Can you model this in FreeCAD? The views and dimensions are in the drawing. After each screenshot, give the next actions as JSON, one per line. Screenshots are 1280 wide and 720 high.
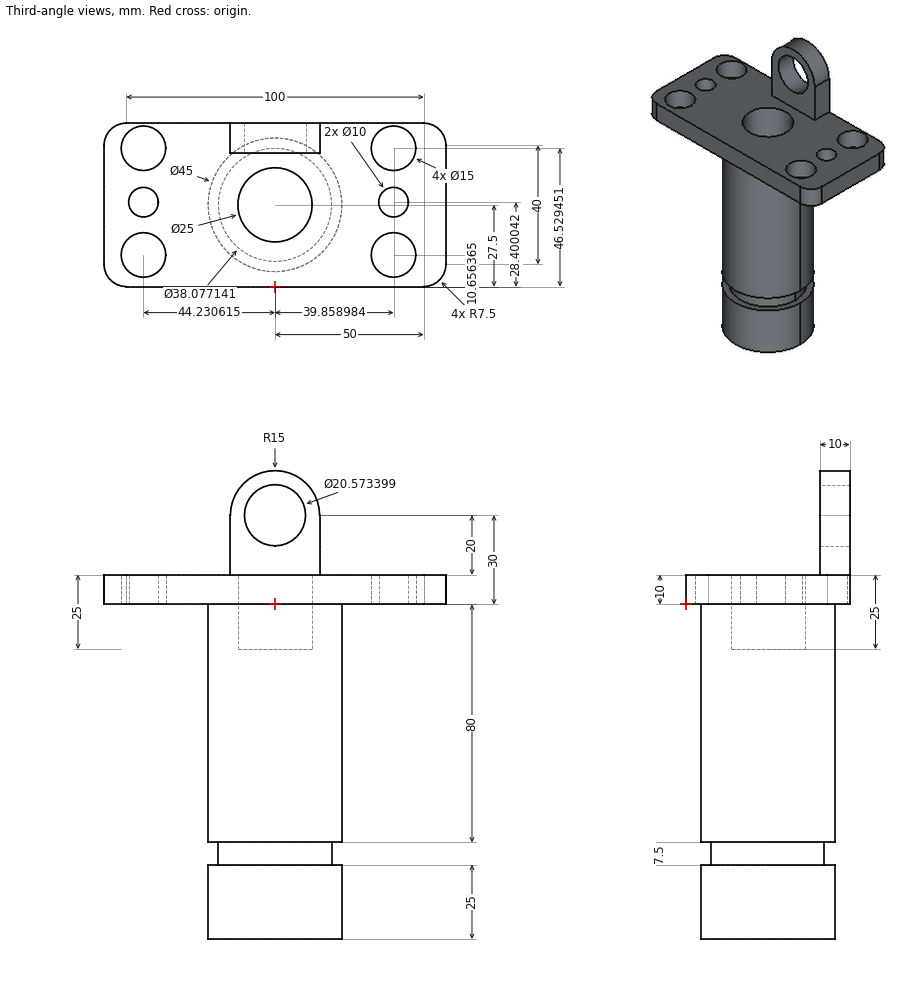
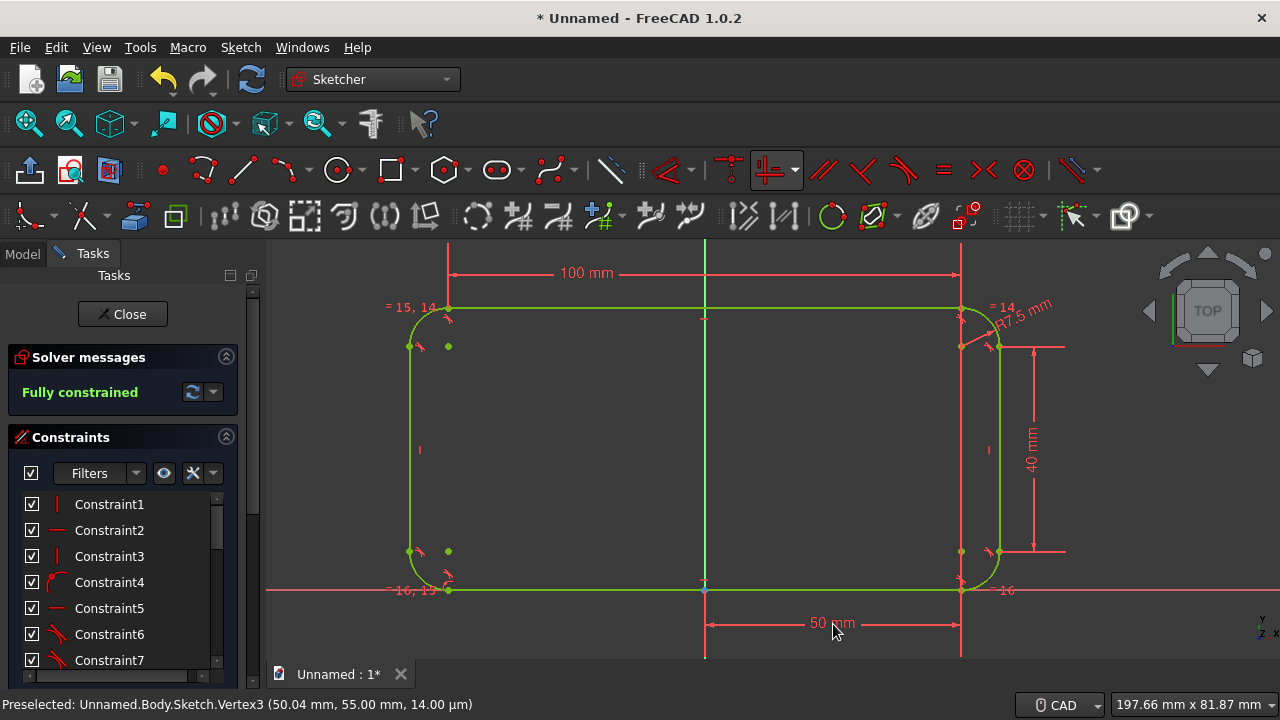
{"action": "left_click", "coordinate": [123, 314]}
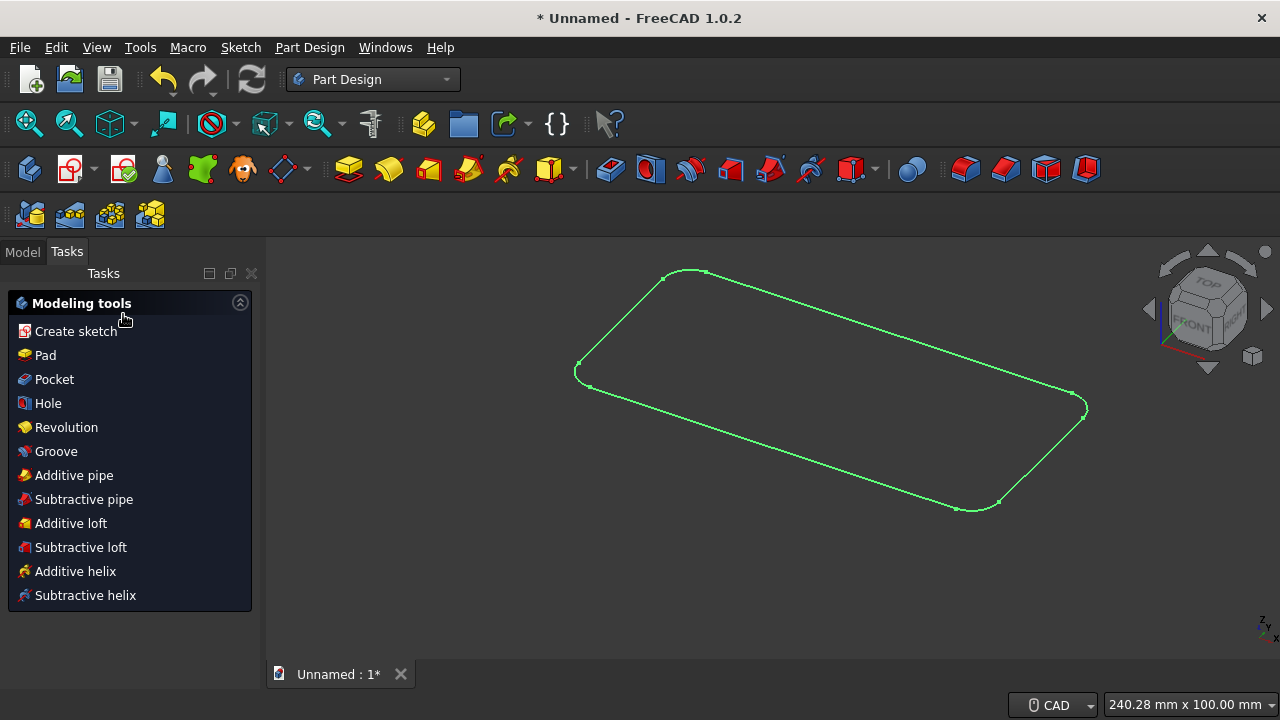
{"action": "left_click", "coordinate": [350, 170]}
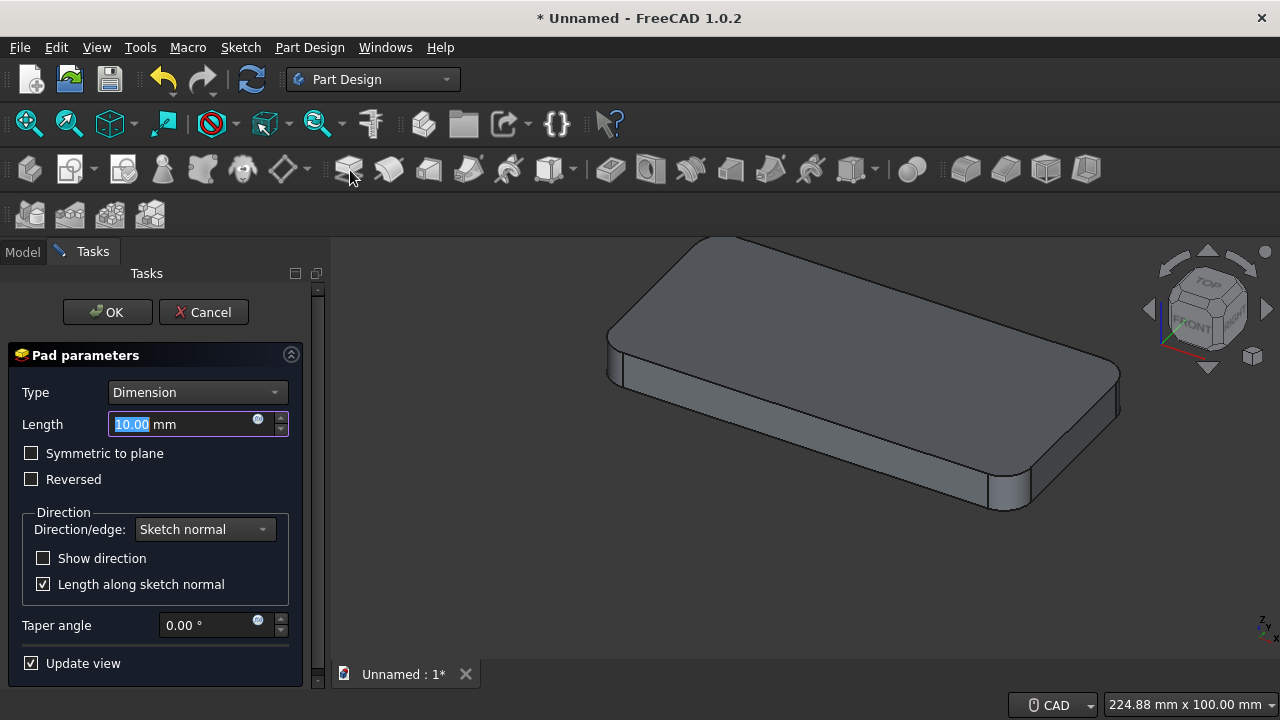
{"action": "type", "text": "10"}
{"action": "key", "text": "Tab"}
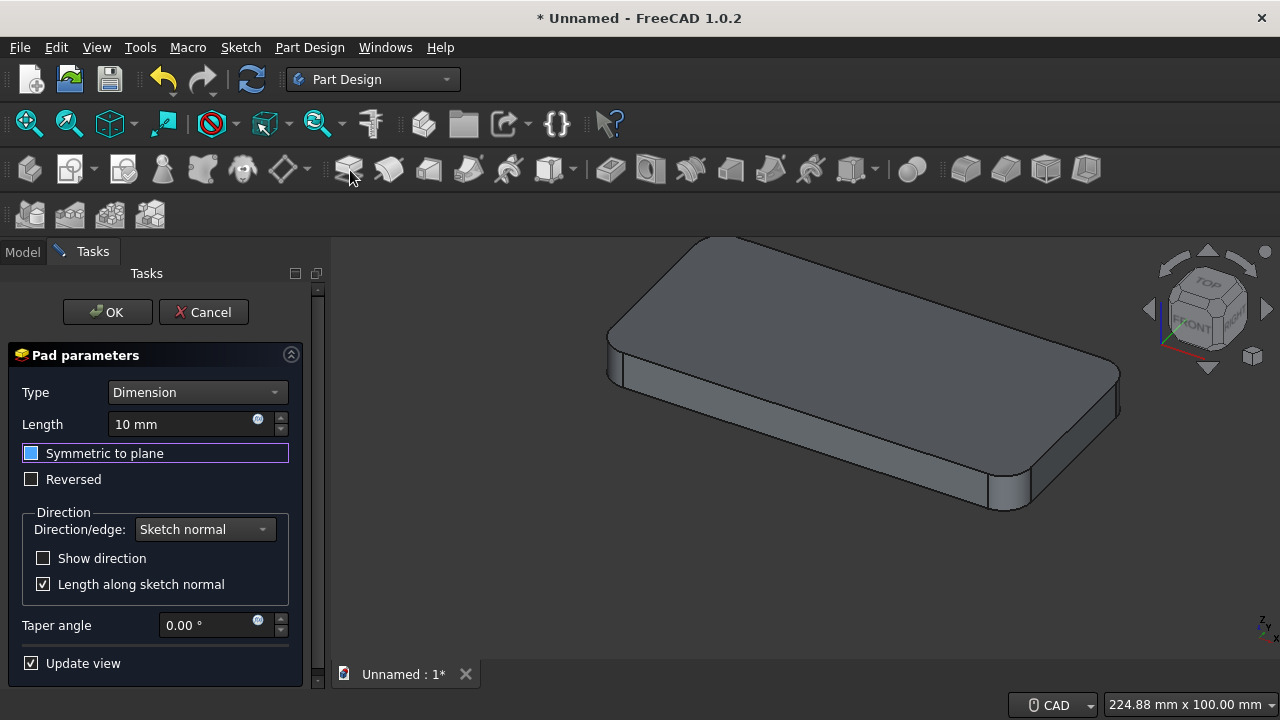
{"action": "left_click", "coordinate": [108, 312]}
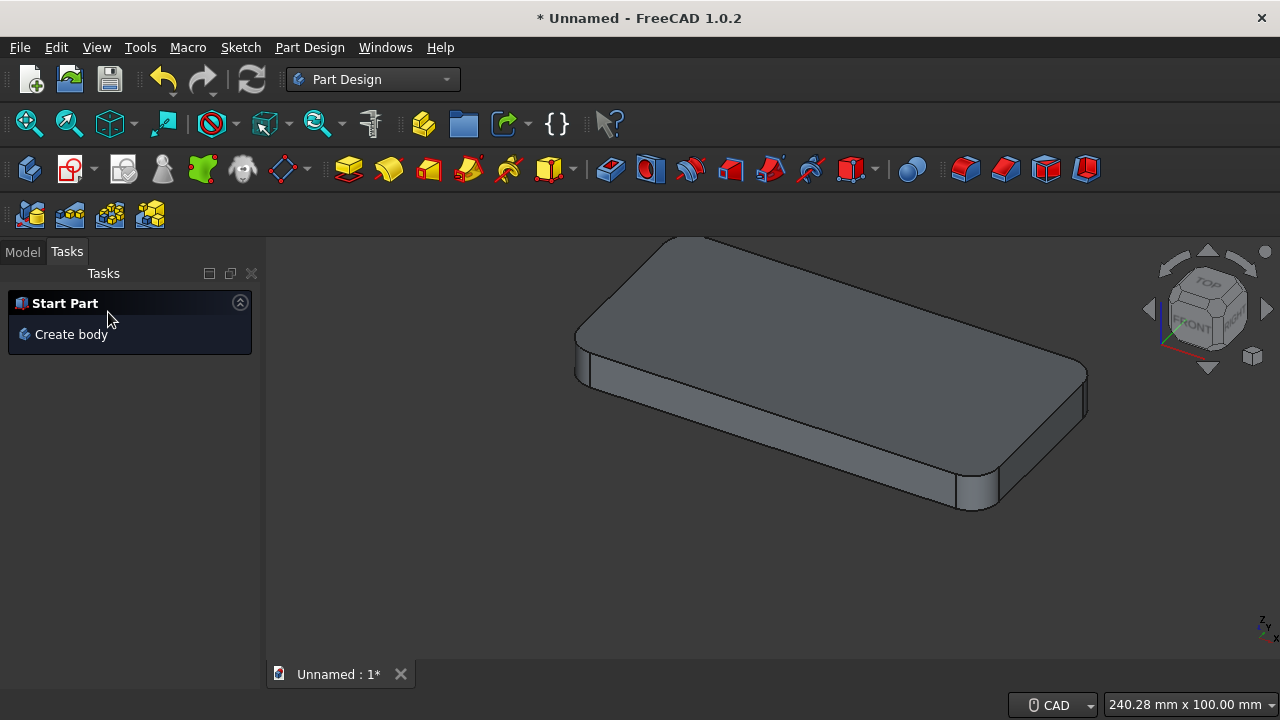
{"action": "left_click", "coordinate": [30, 124]}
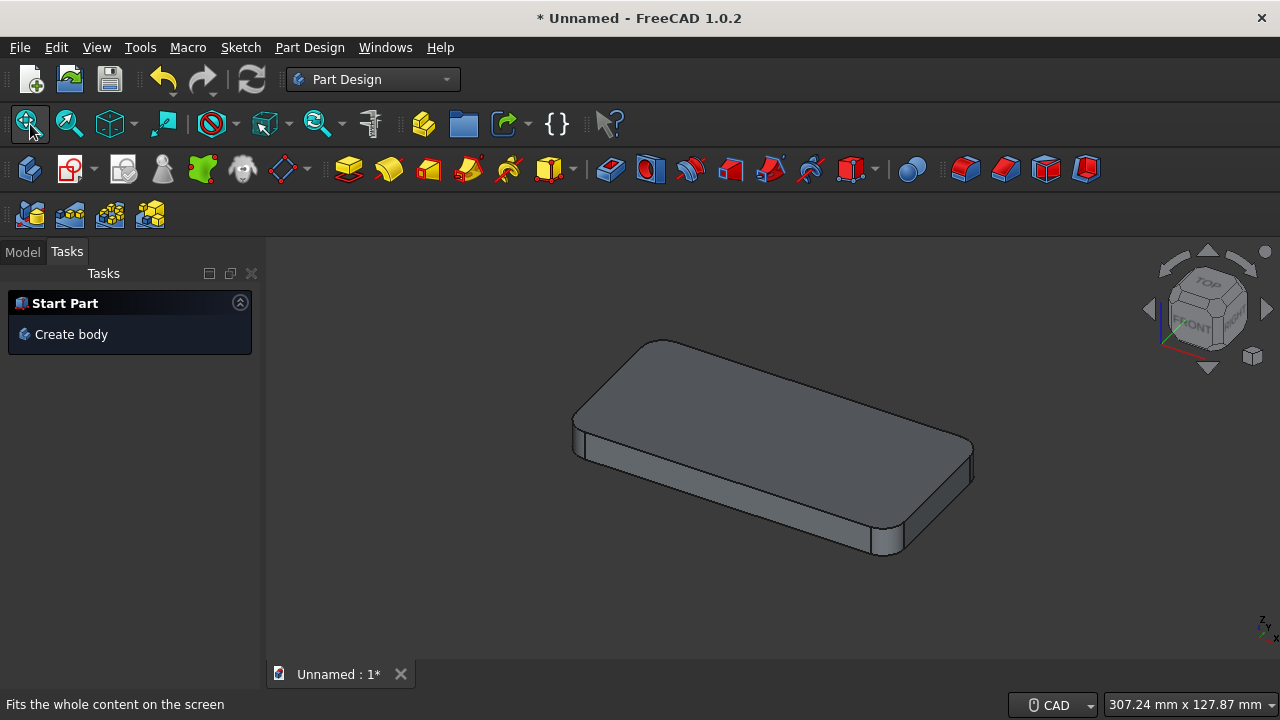
{"action": "key", "text": "5"}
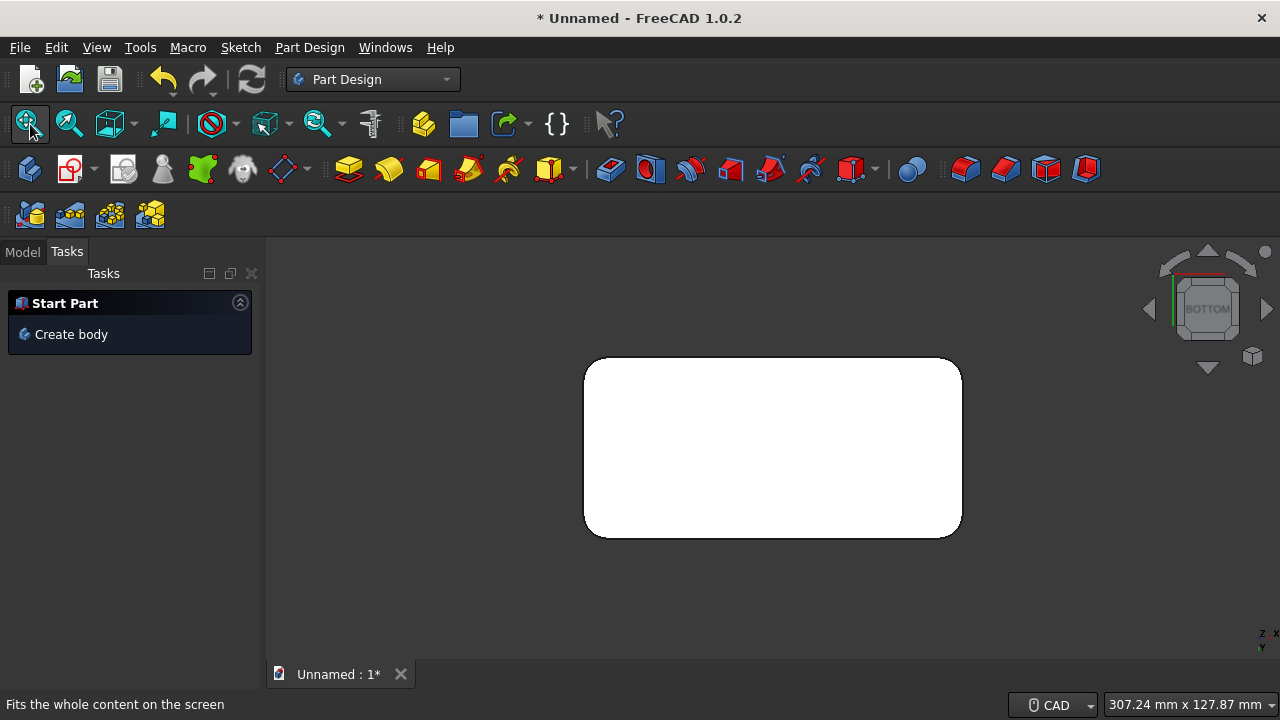
{"action": "left_click", "coordinate": [30, 124]}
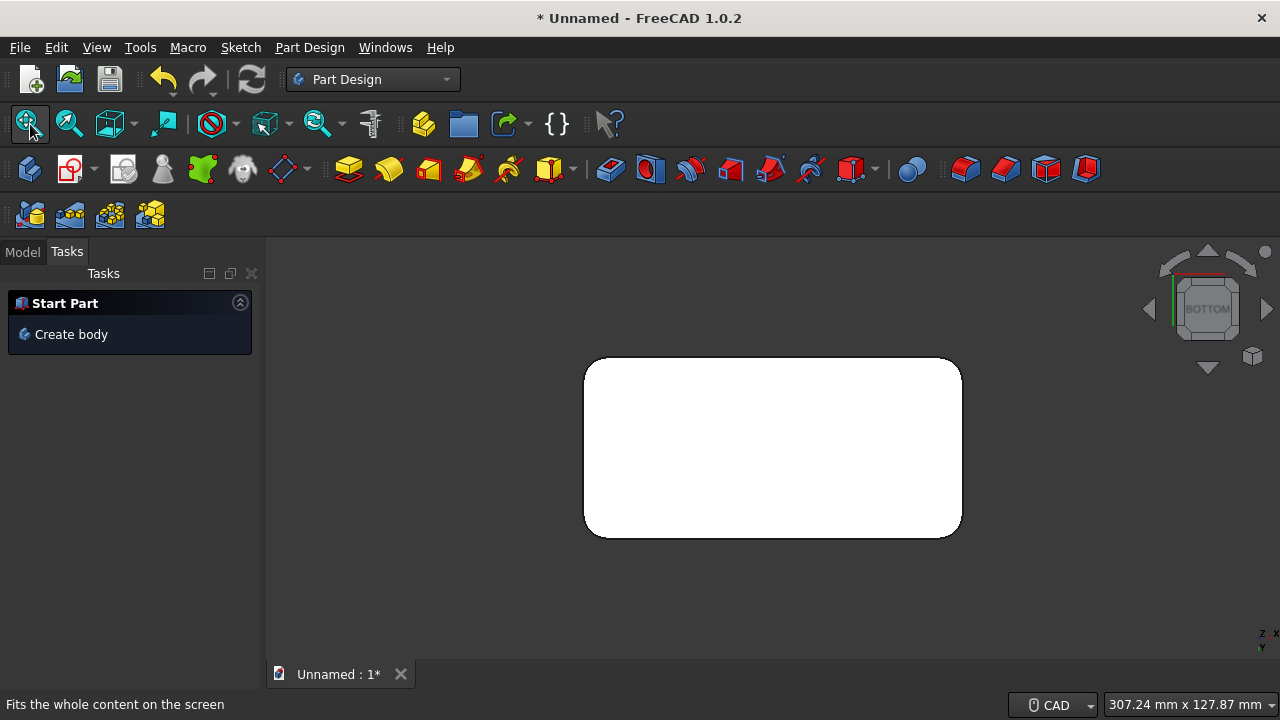
{"action": "left_click", "coordinate": [827, 447]}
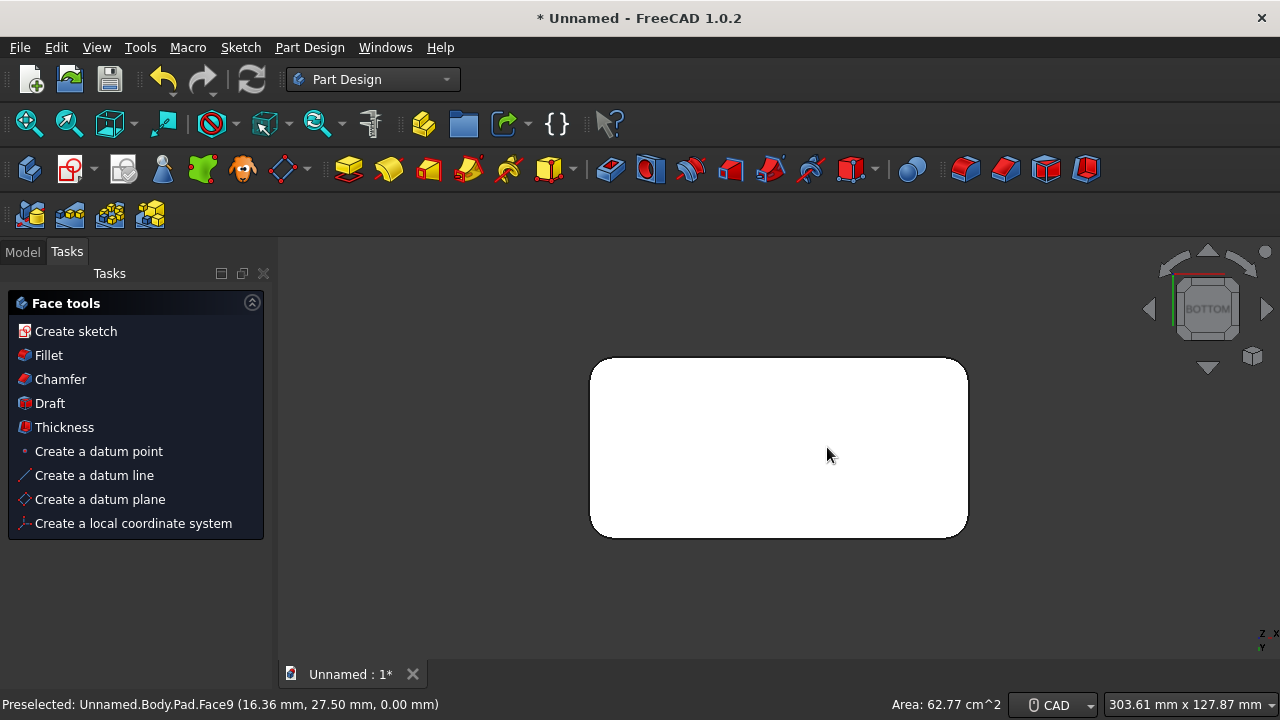
{"action": "left_click", "coordinate": [70, 170]}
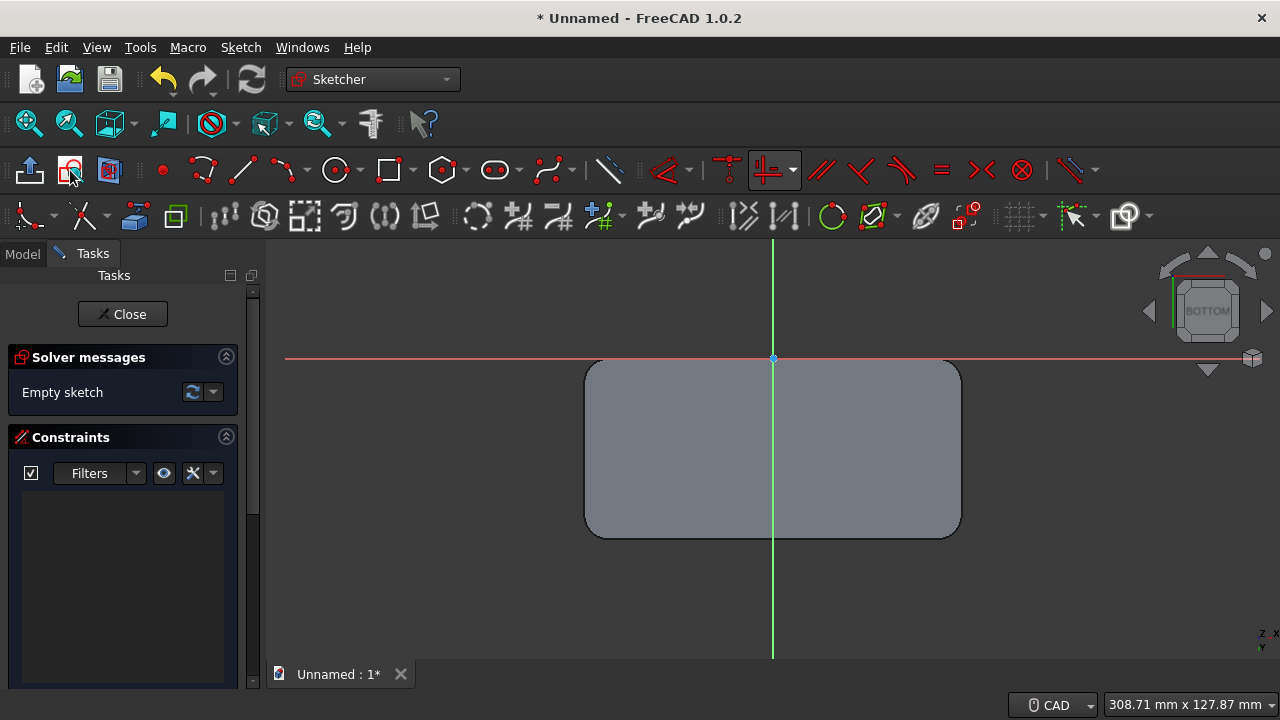
{"action": "scroll", "coordinate": [912, 424], "scroll_direction": "up", "scroll_amount": 2}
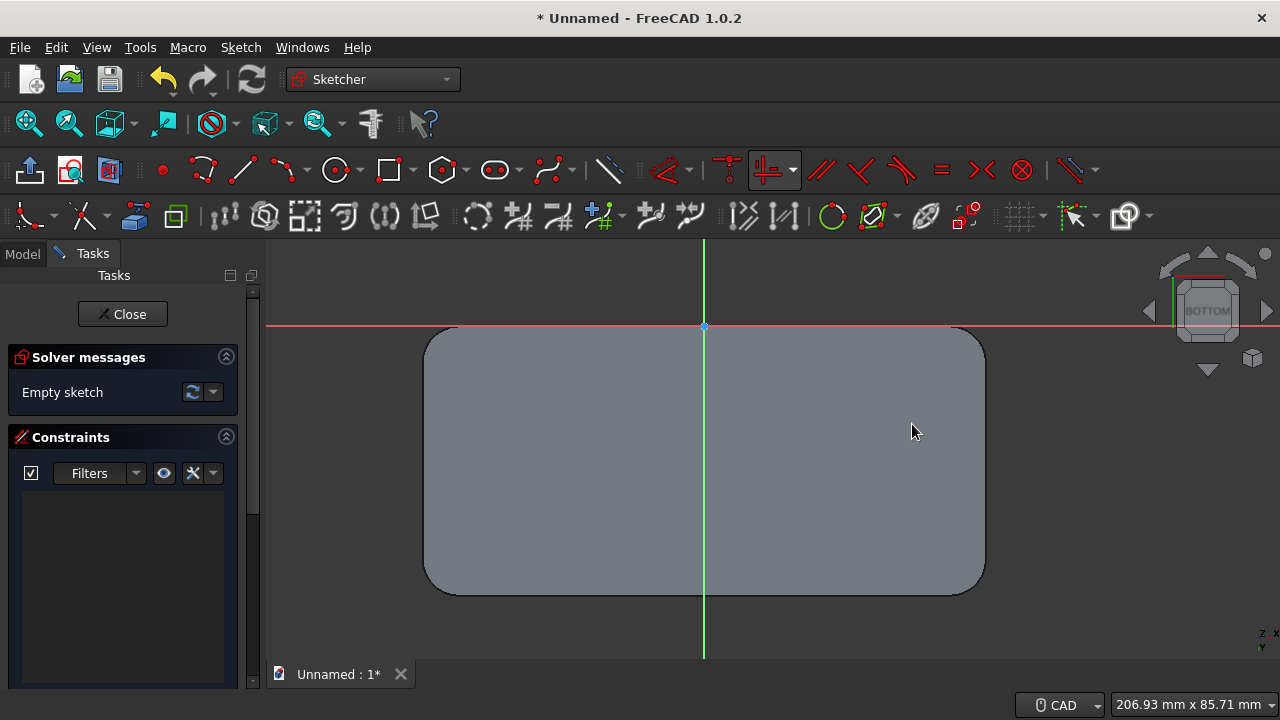
{"action": "left_click", "coordinate": [336, 170]}